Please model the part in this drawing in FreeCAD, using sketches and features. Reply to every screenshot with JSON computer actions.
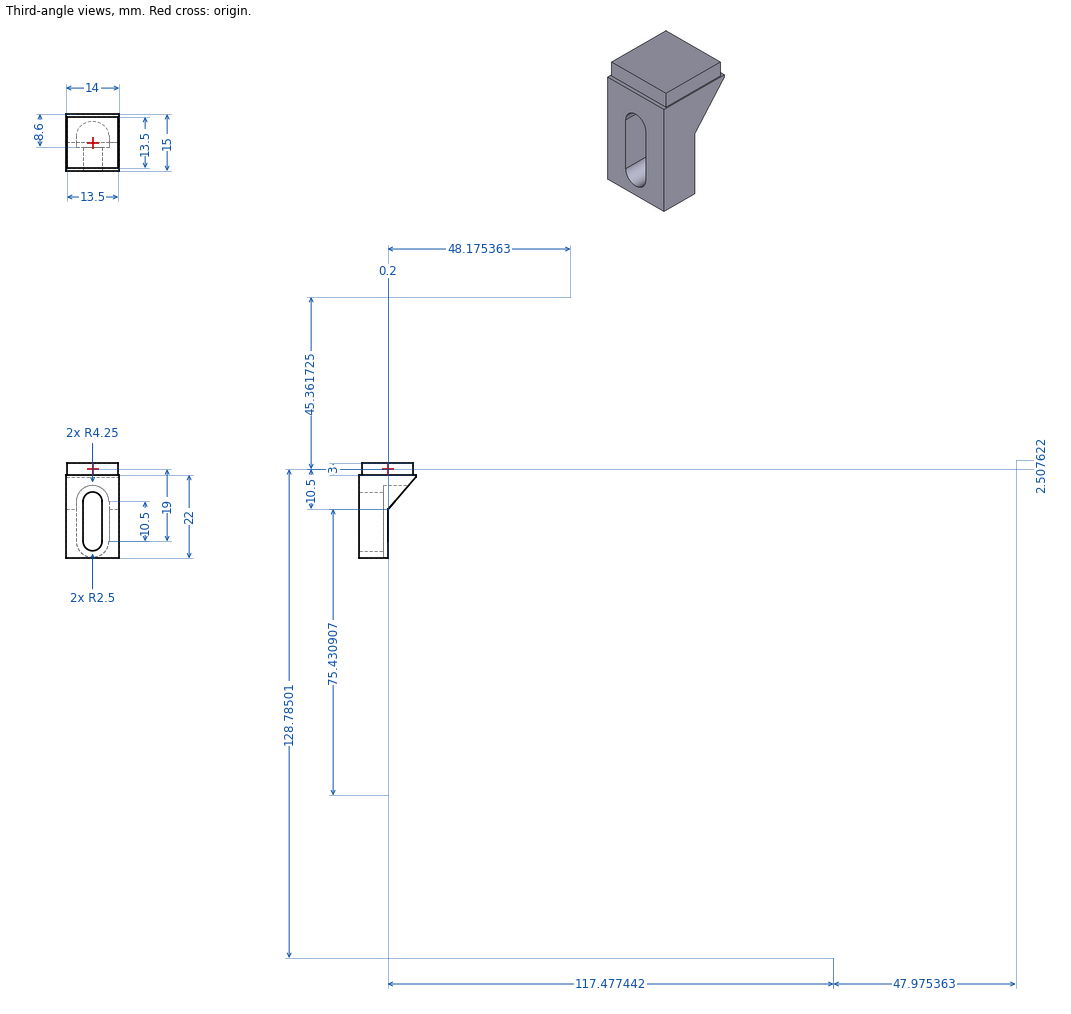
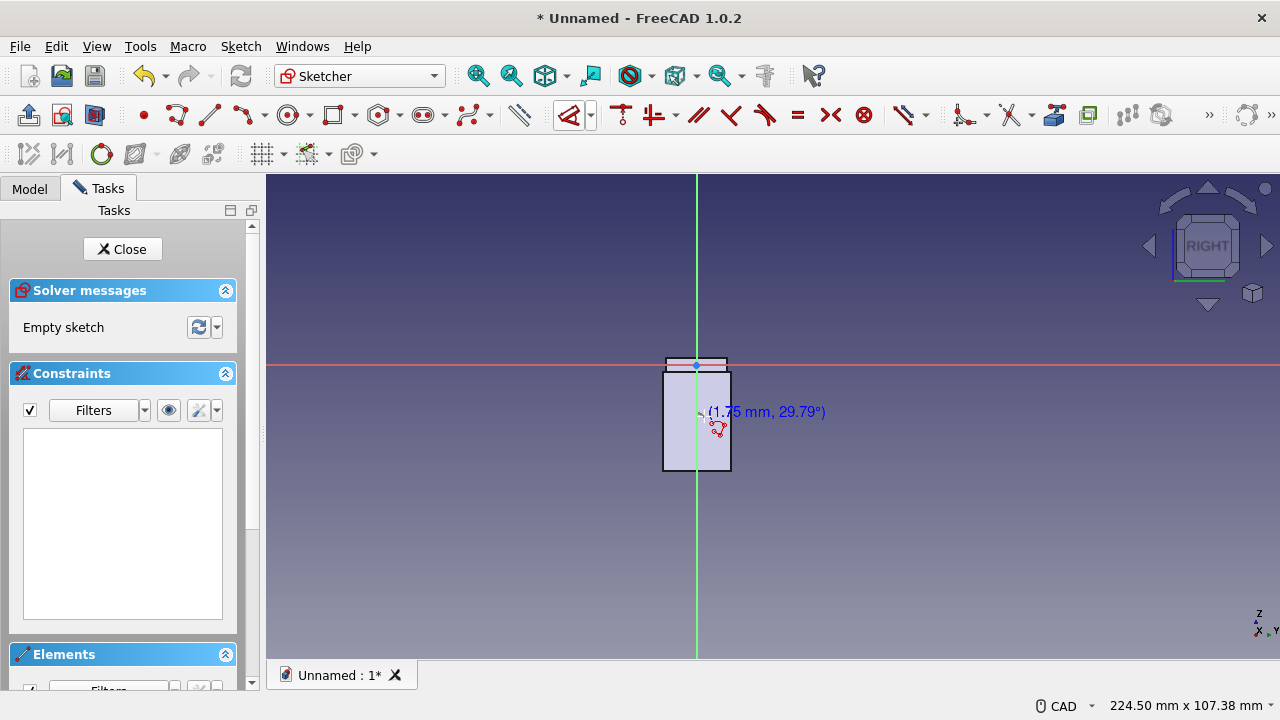
{"action": "scroll", "coordinate": [492, 337], "scroll_direction": "down", "scroll_amount": 5}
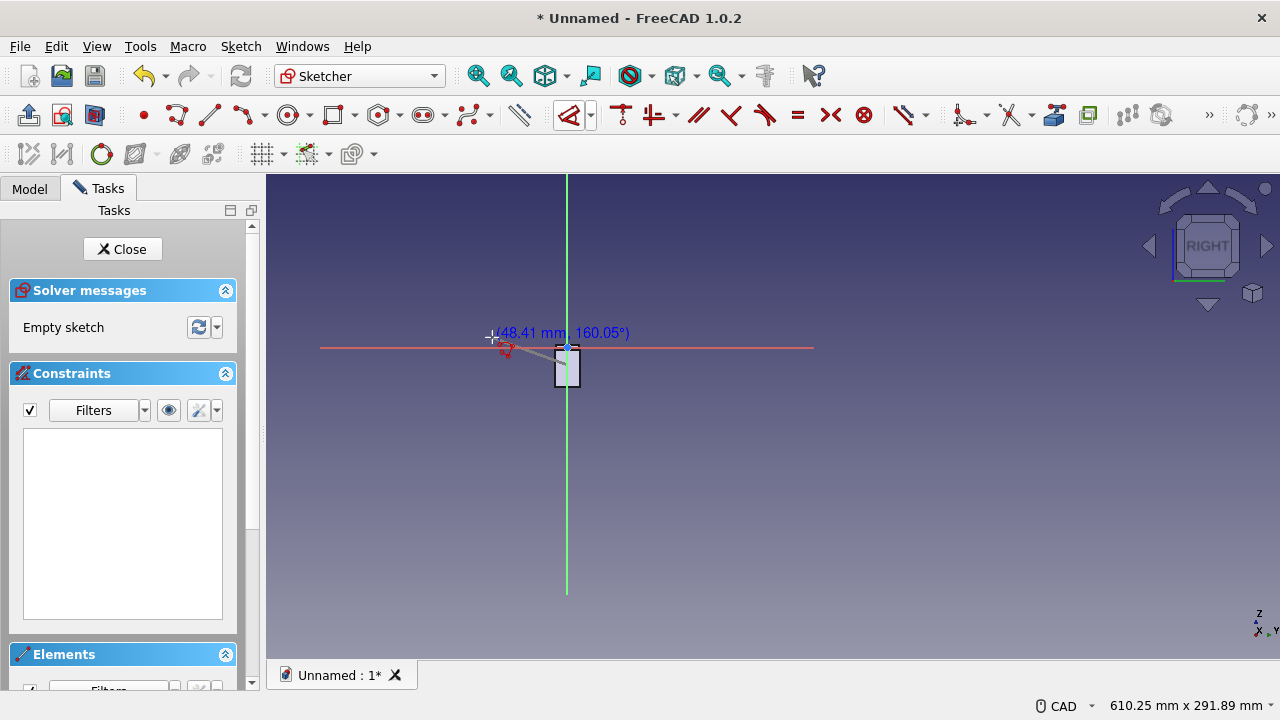
{"action": "scroll", "coordinate": [568, 490], "scroll_direction": "up", "scroll_amount": 20}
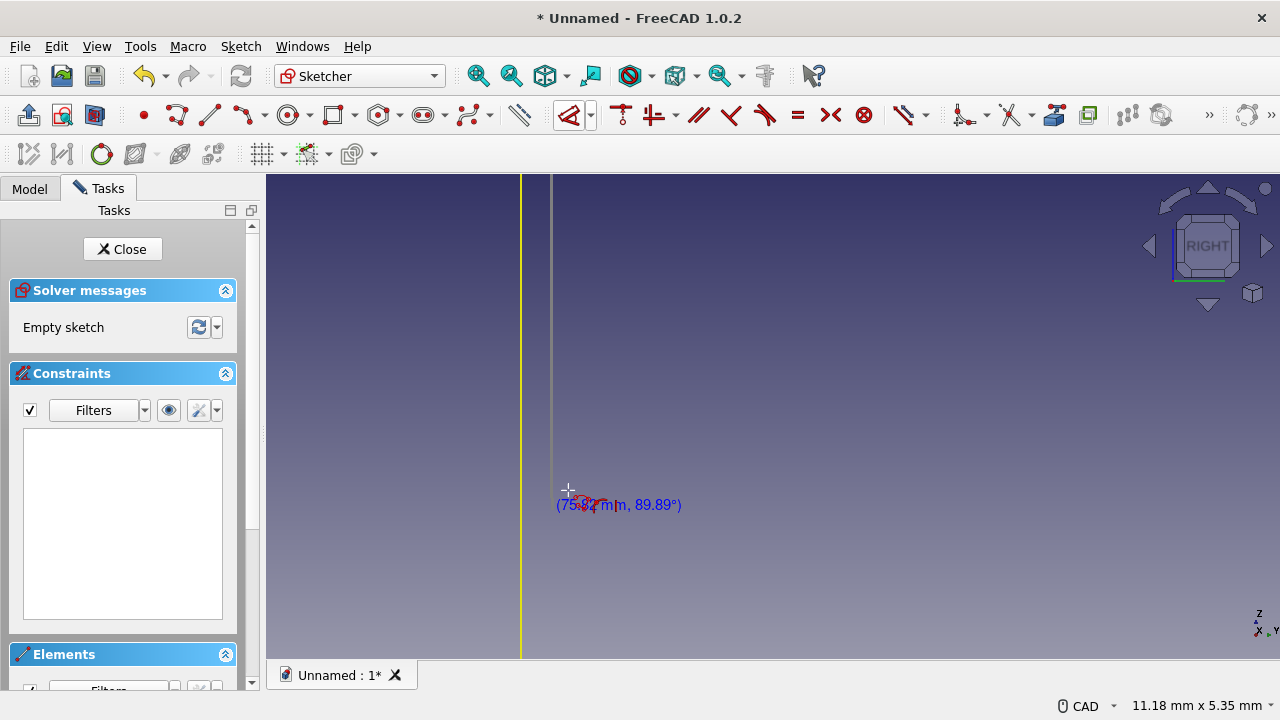
{"action": "left_click", "coordinate": [539, 474]}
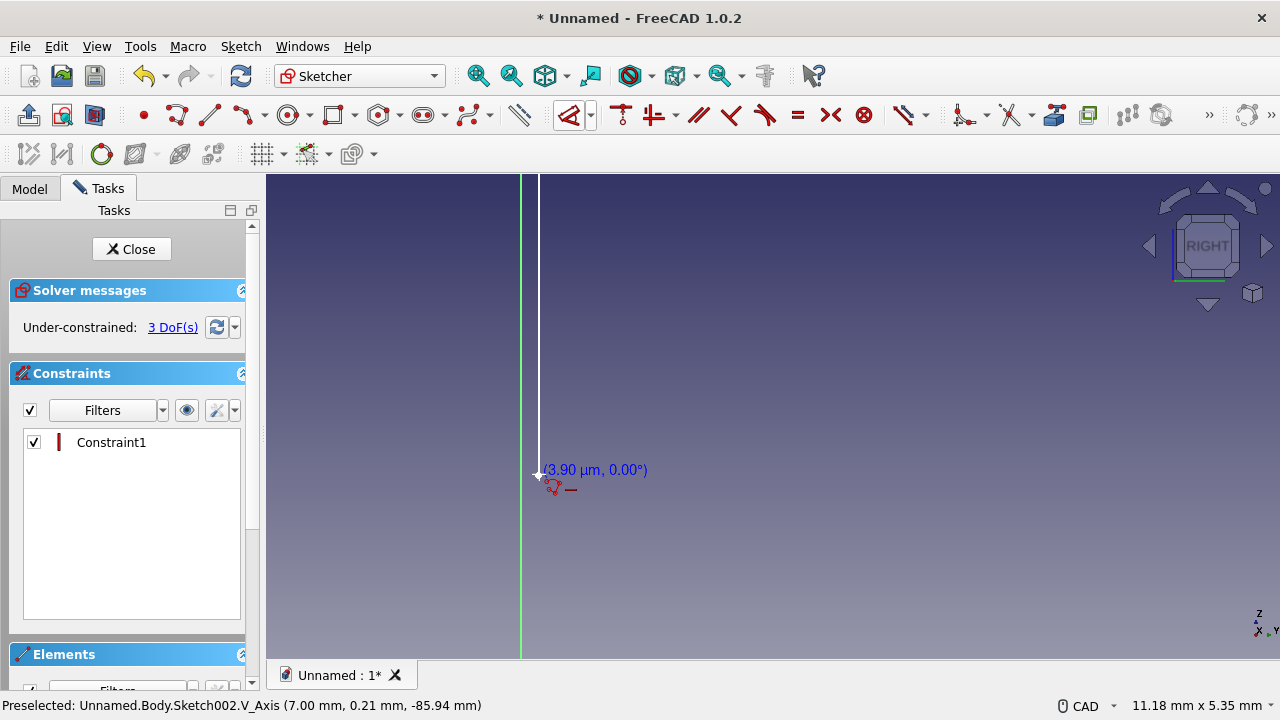
{"action": "scroll", "coordinate": [704, 416], "scroll_direction": "down", "scroll_amount": 15}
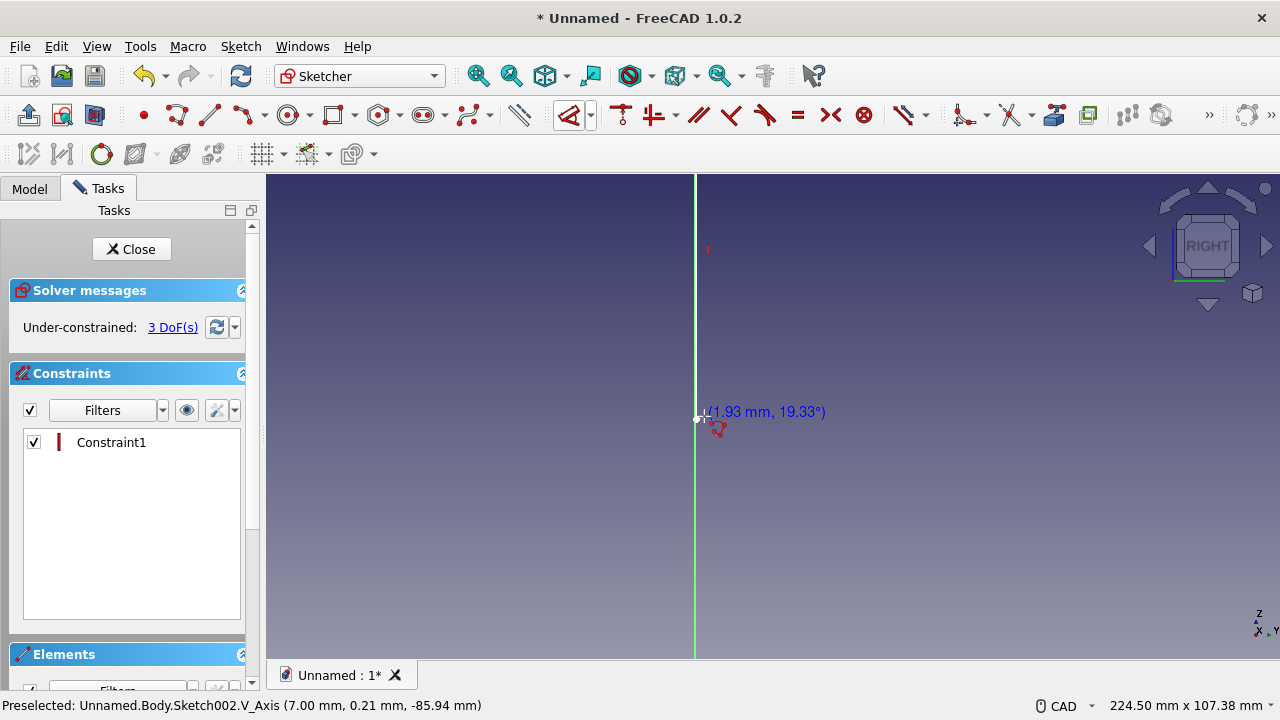
{"action": "scroll", "coordinate": [492, 531], "scroll_direction": "down", "scroll_amount": 5}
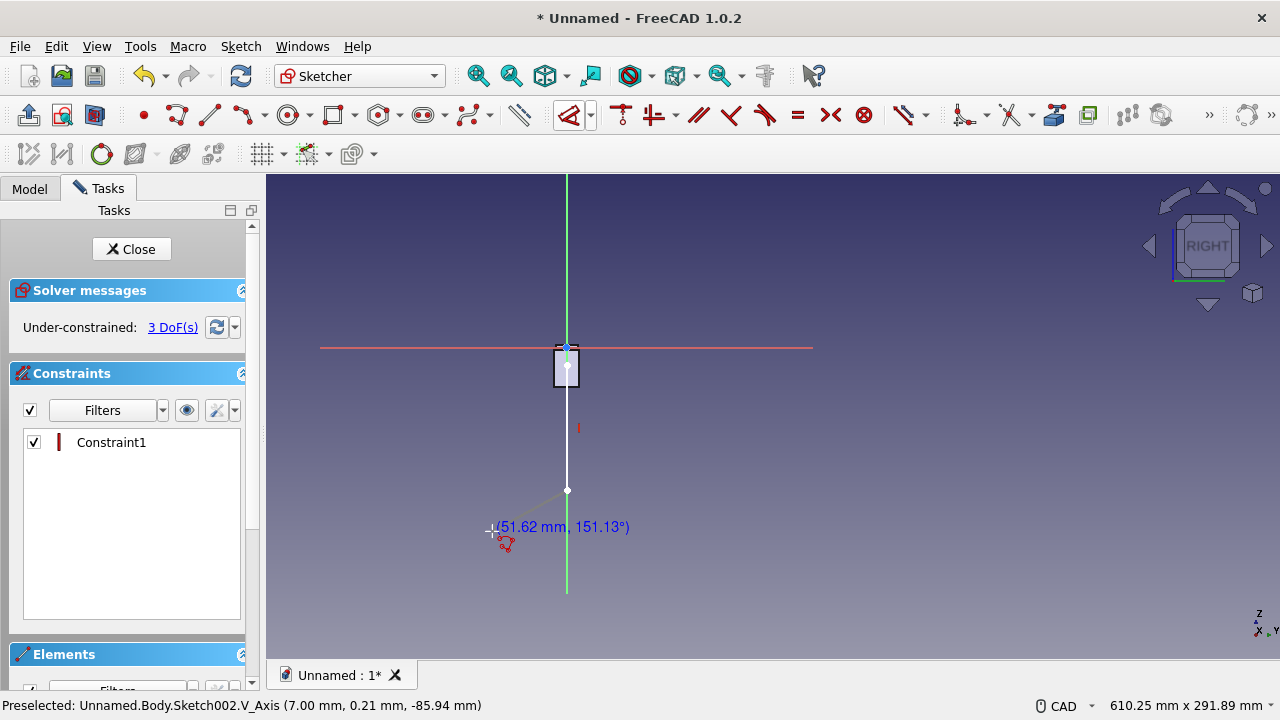
{"action": "left_click", "coordinate": [762, 562]}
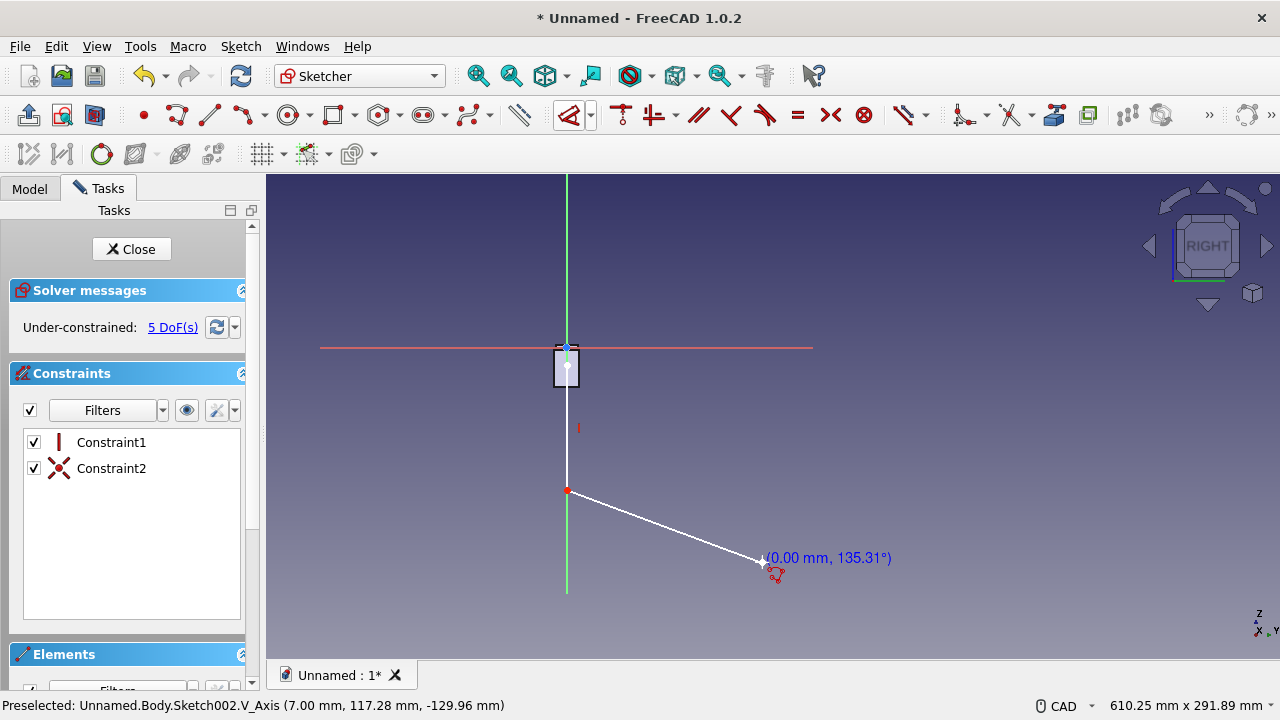
{"action": "scroll", "coordinate": [842, 343], "scroll_direction": "up", "scroll_amount": 7}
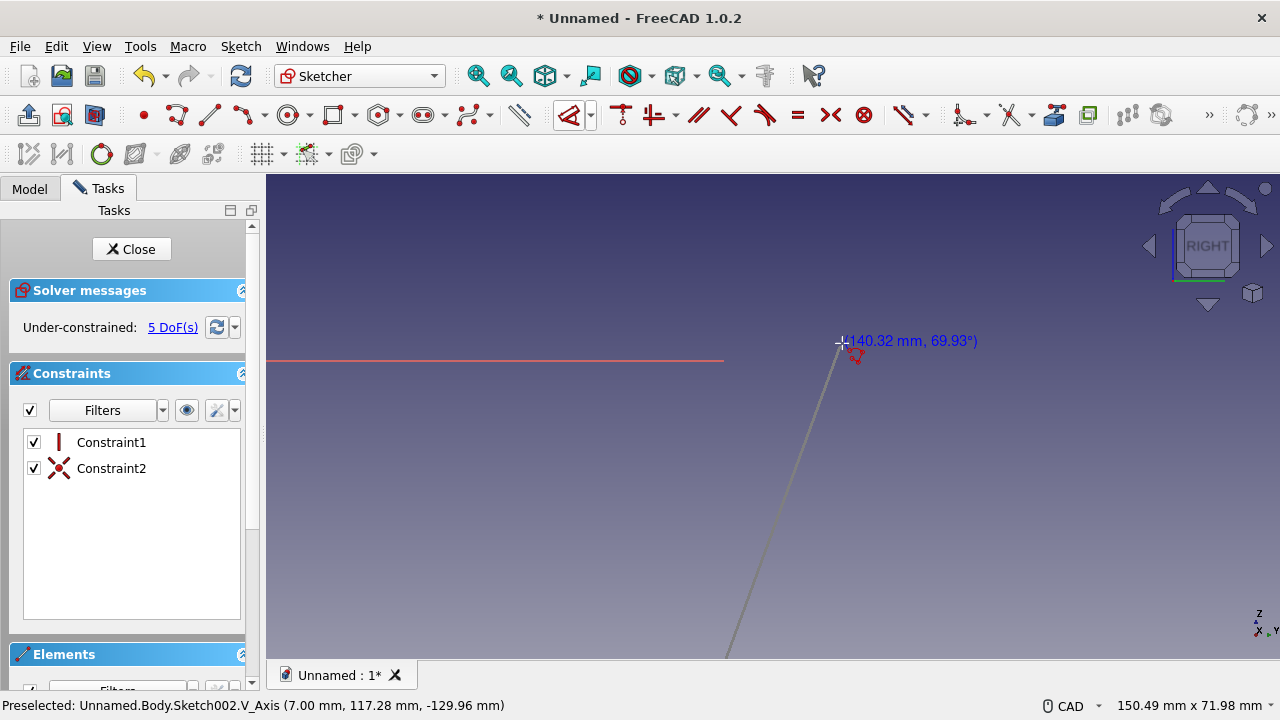
{"action": "left_click", "coordinate": [840, 344]}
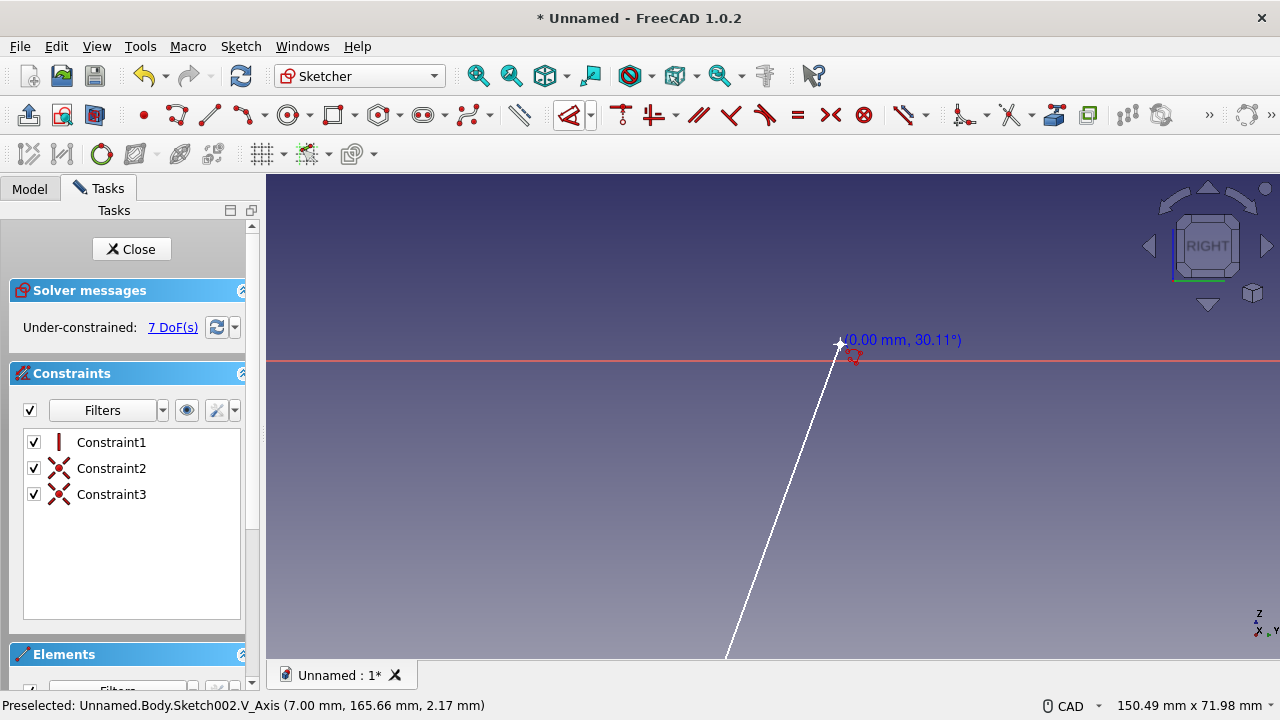
{"action": "scroll", "coordinate": [843, 343], "scroll_direction": "down", "scroll_amount": 7}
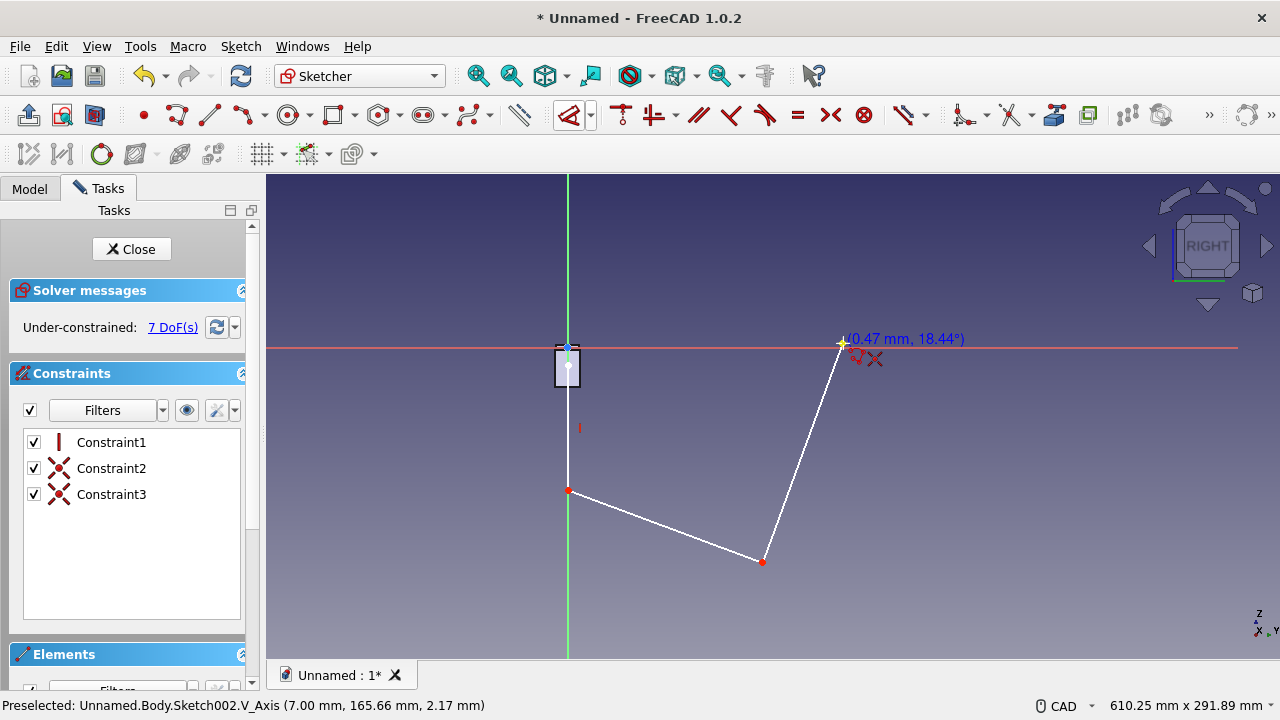
{"action": "left_click", "coordinate": [648, 272]}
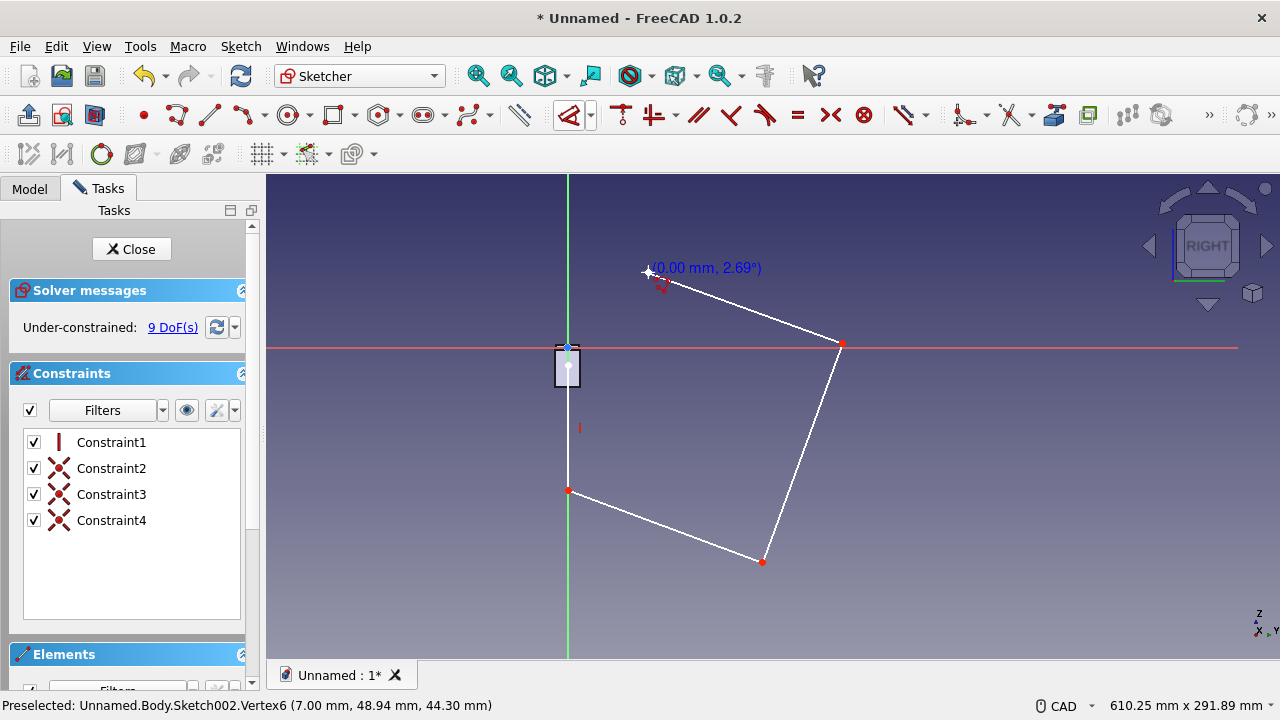
{"action": "scroll", "coordinate": [568, 365], "scroll_direction": "up", "scroll_amount": 20}